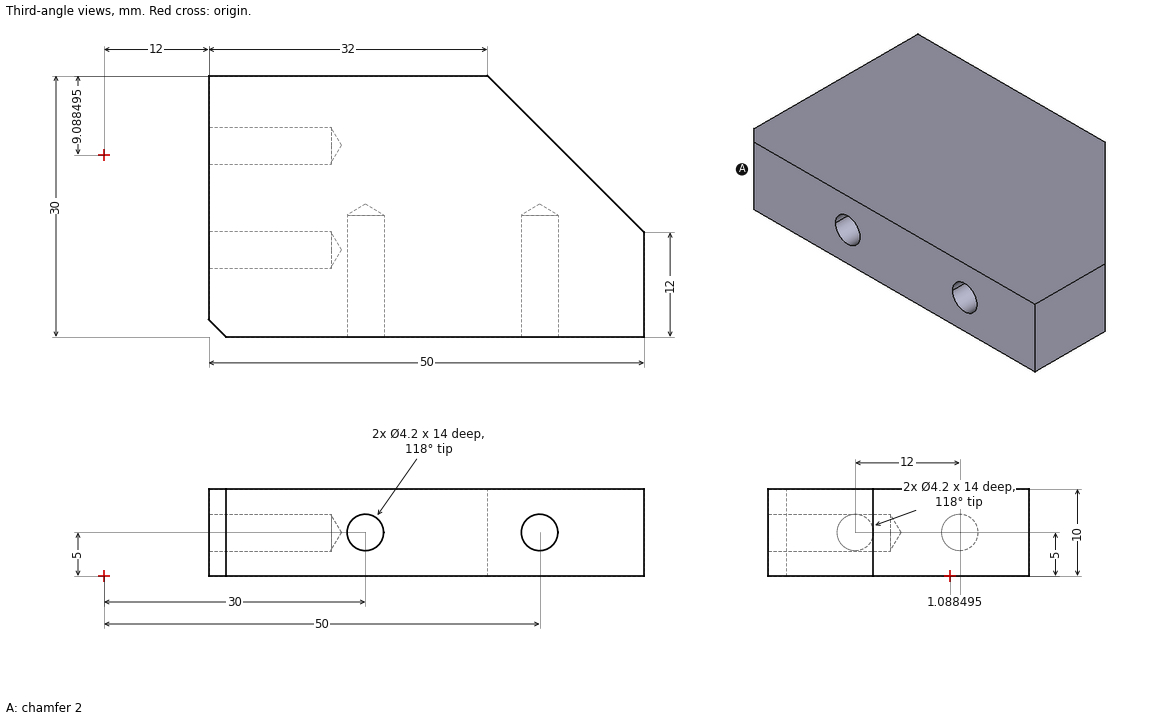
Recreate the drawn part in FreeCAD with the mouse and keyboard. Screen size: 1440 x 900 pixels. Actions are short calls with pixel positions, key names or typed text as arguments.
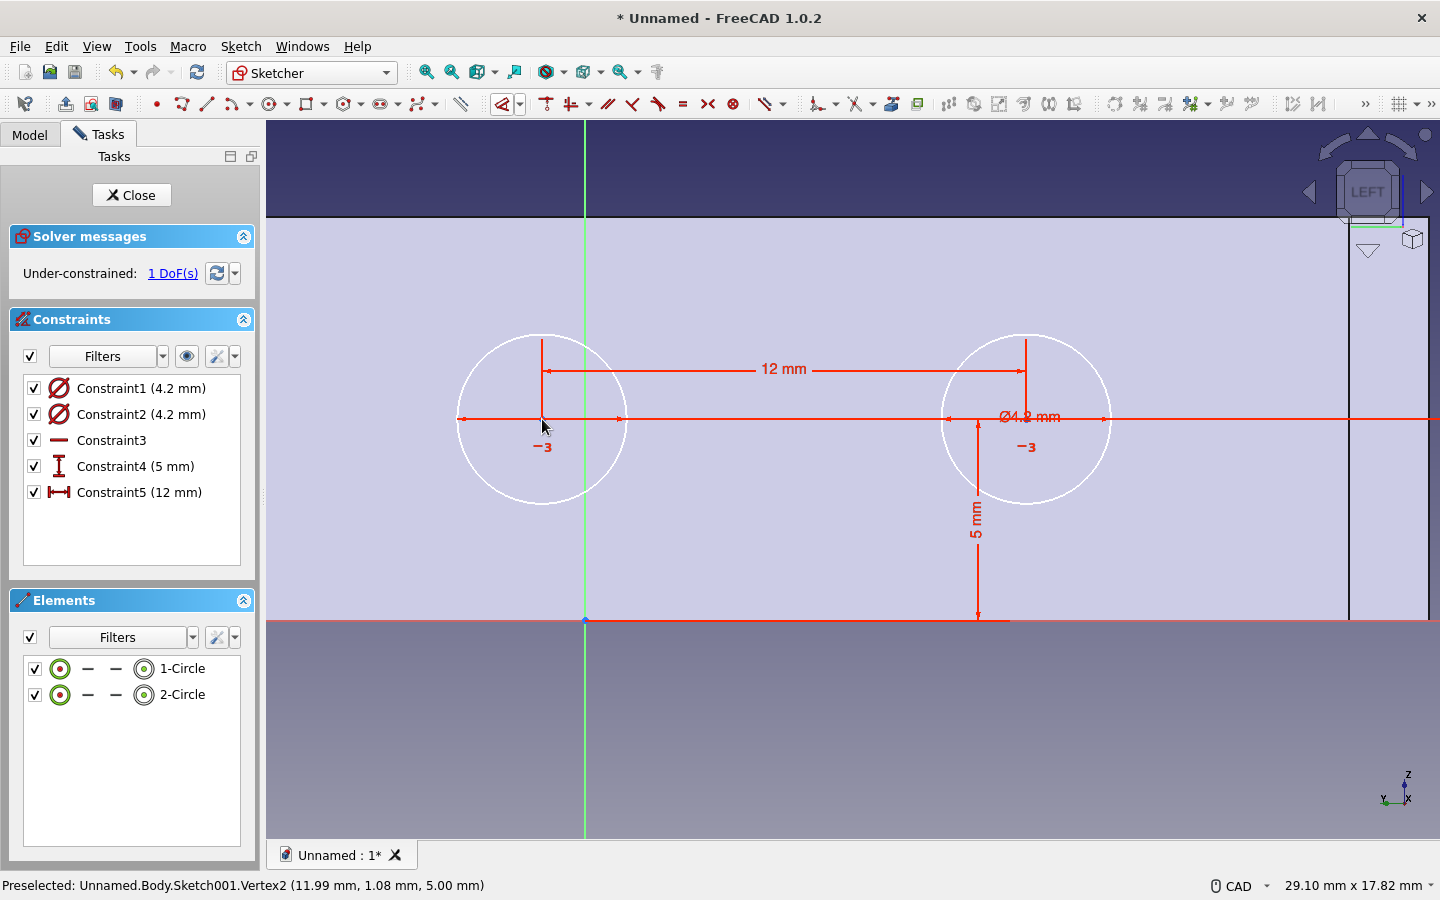
click(542, 419)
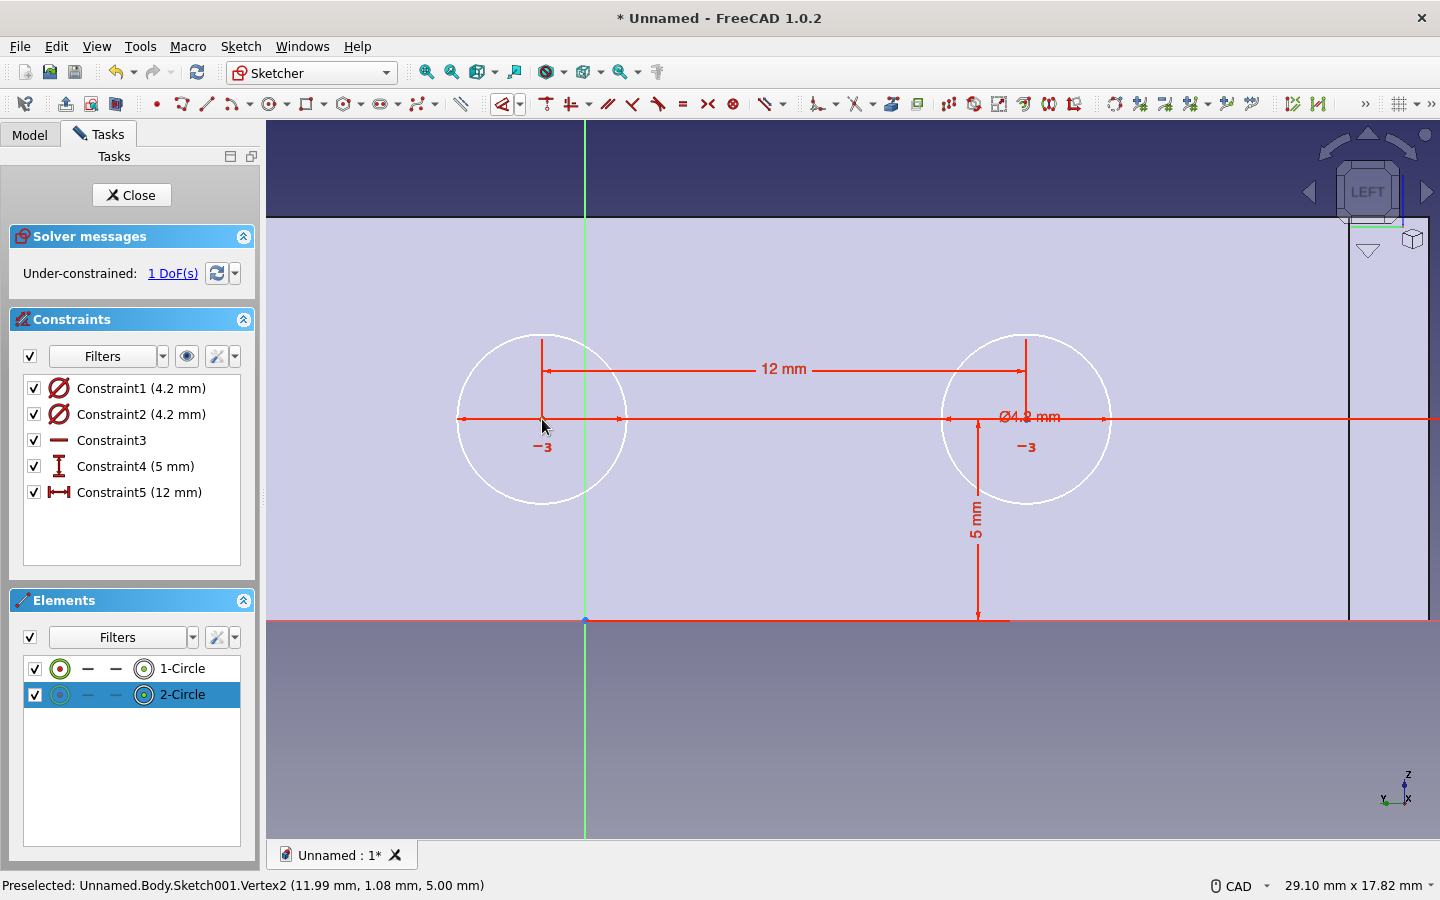
click(520, 104)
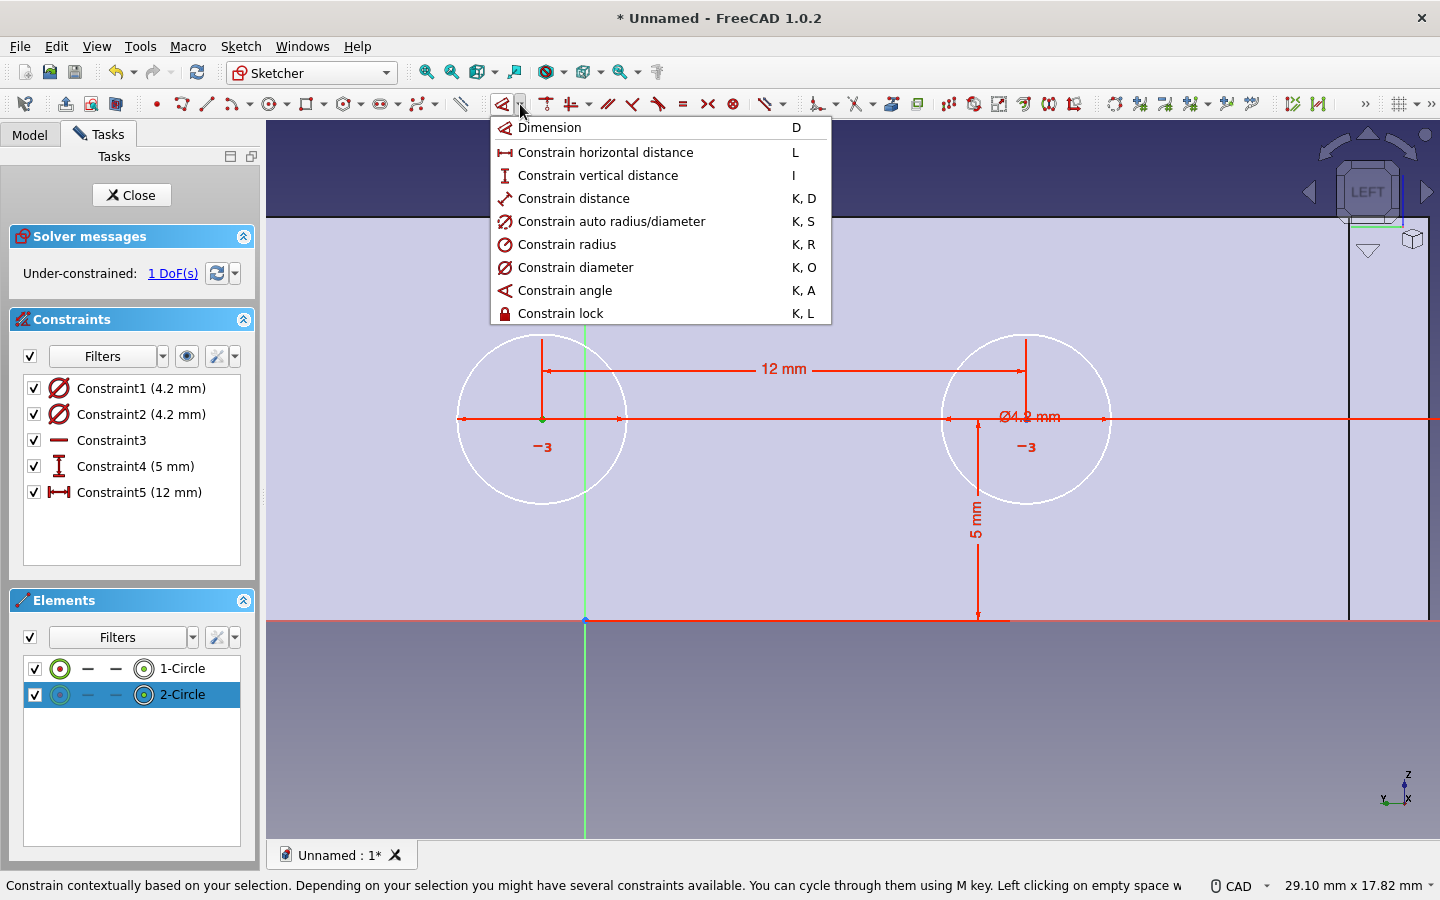
click(661, 152)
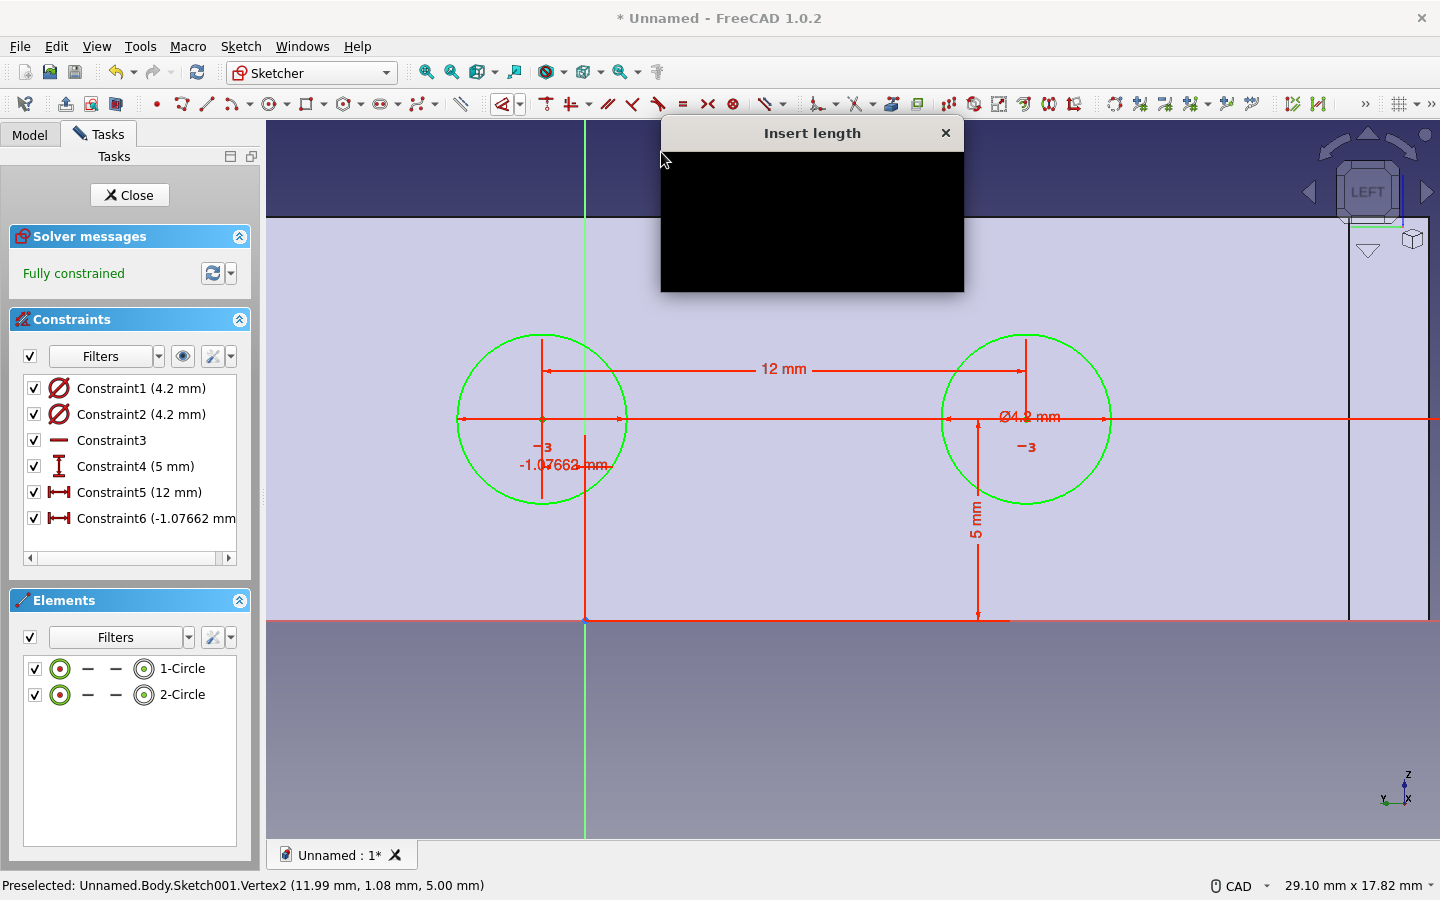
text(-1.088495)
key(Return)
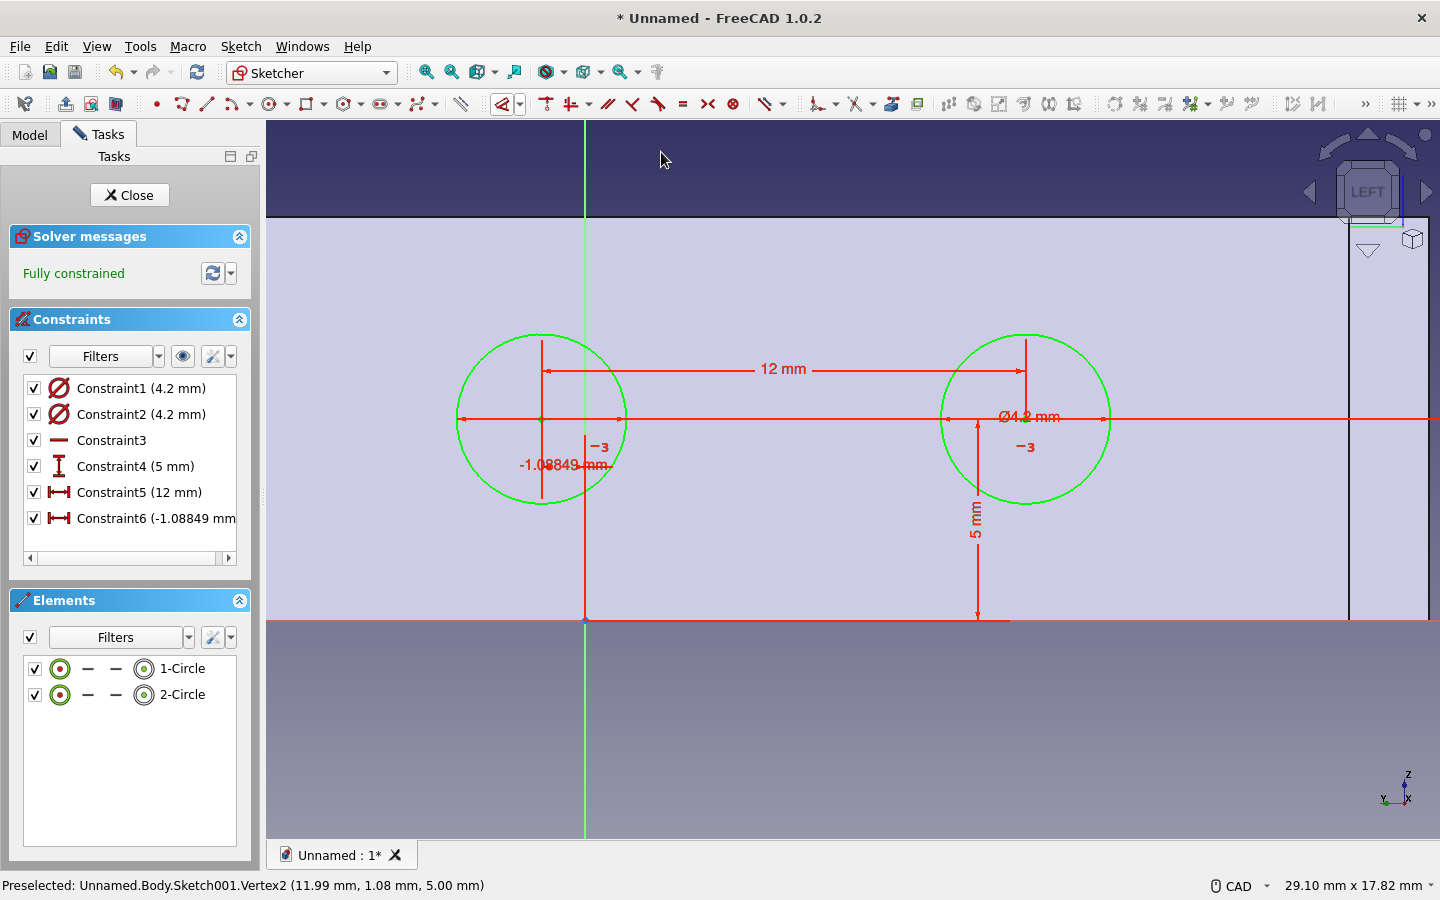
click(130, 195)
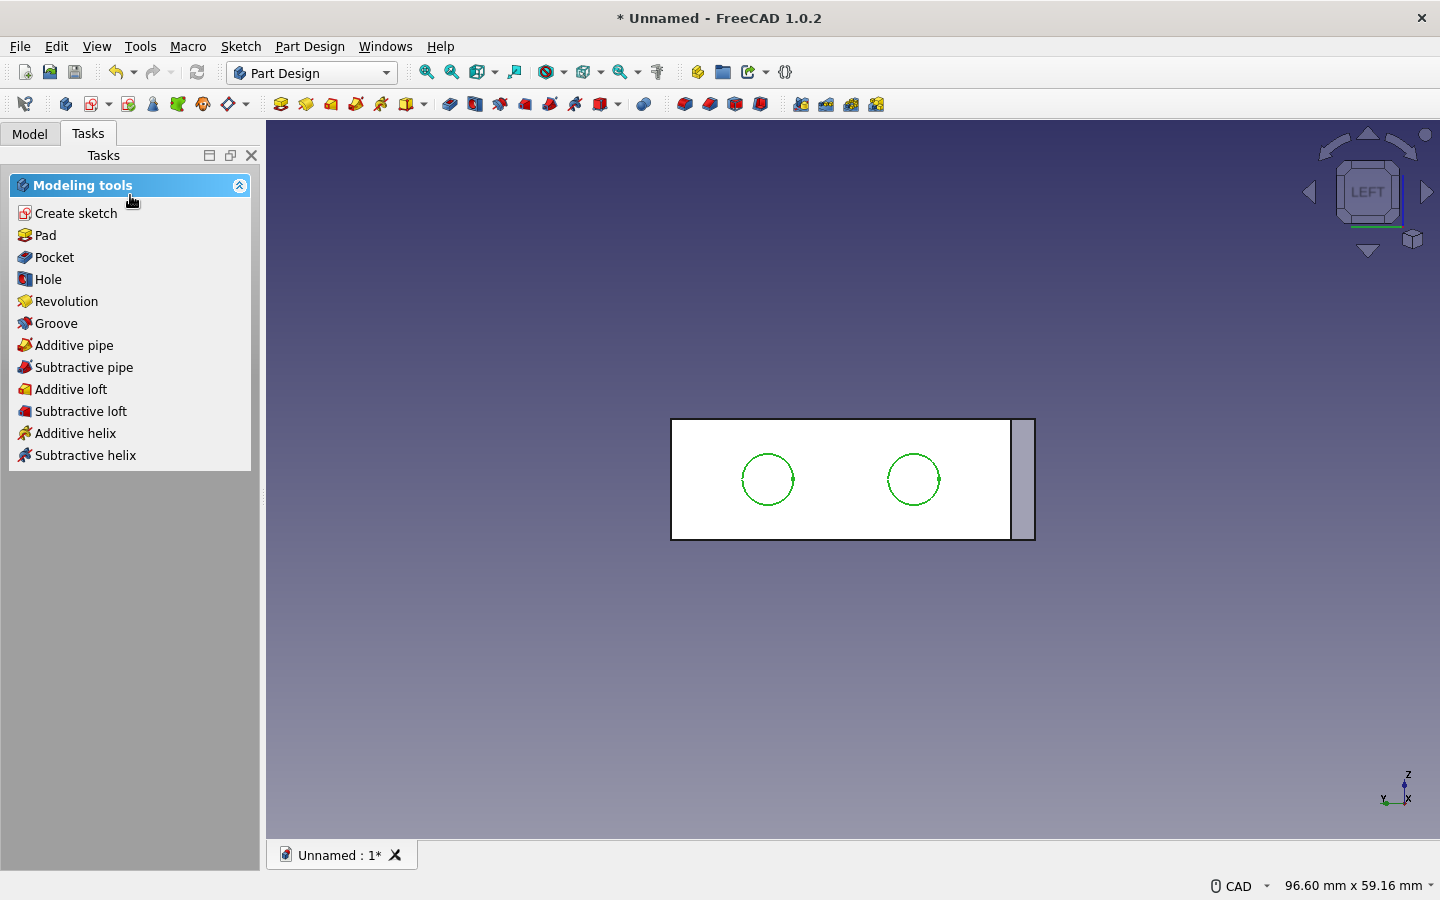
click(475, 104)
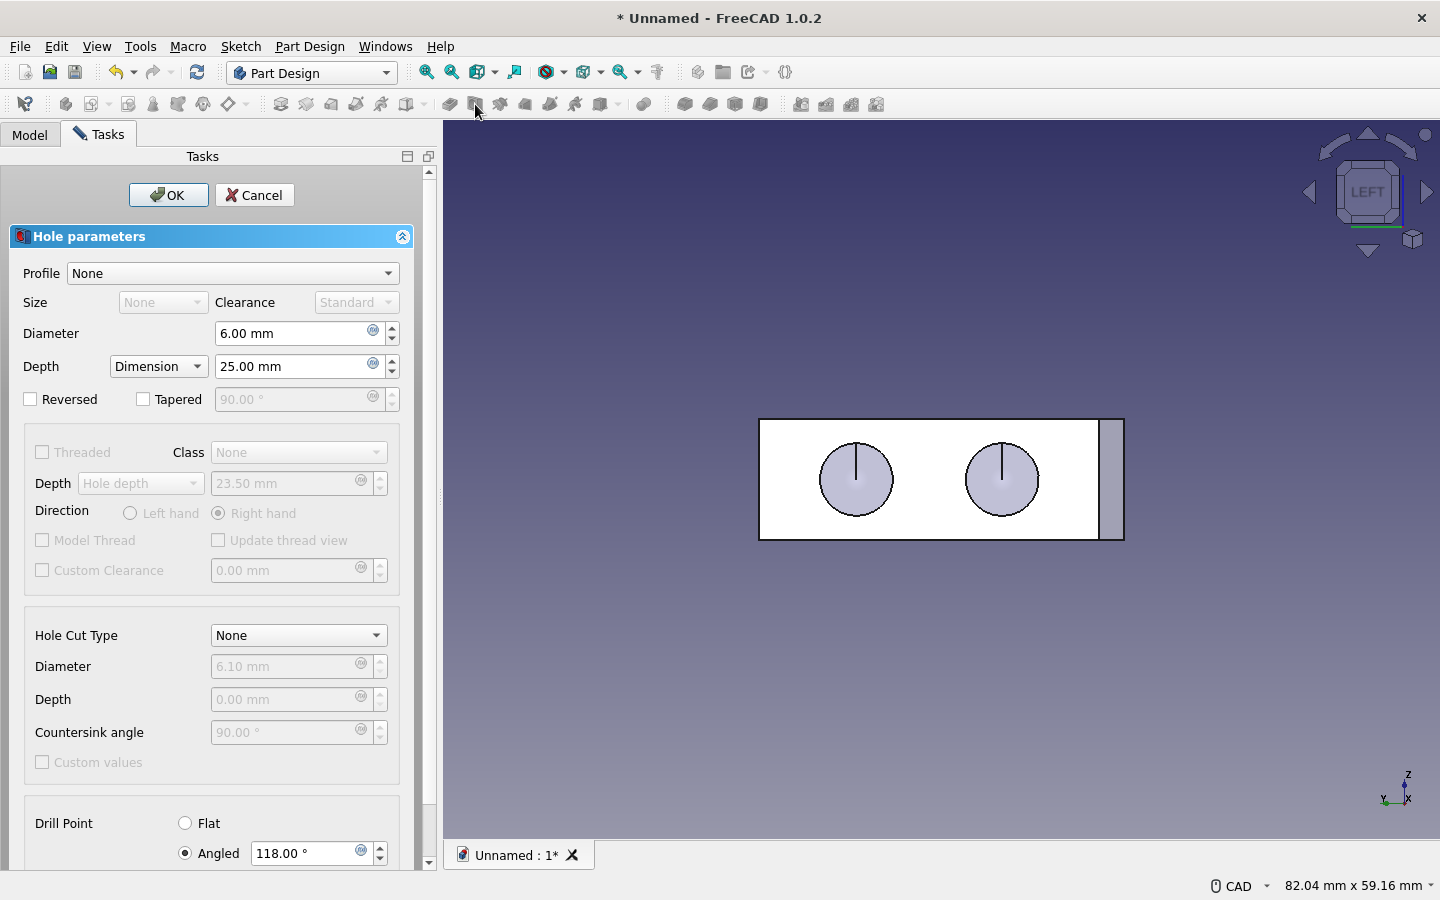
triple_click(300, 334)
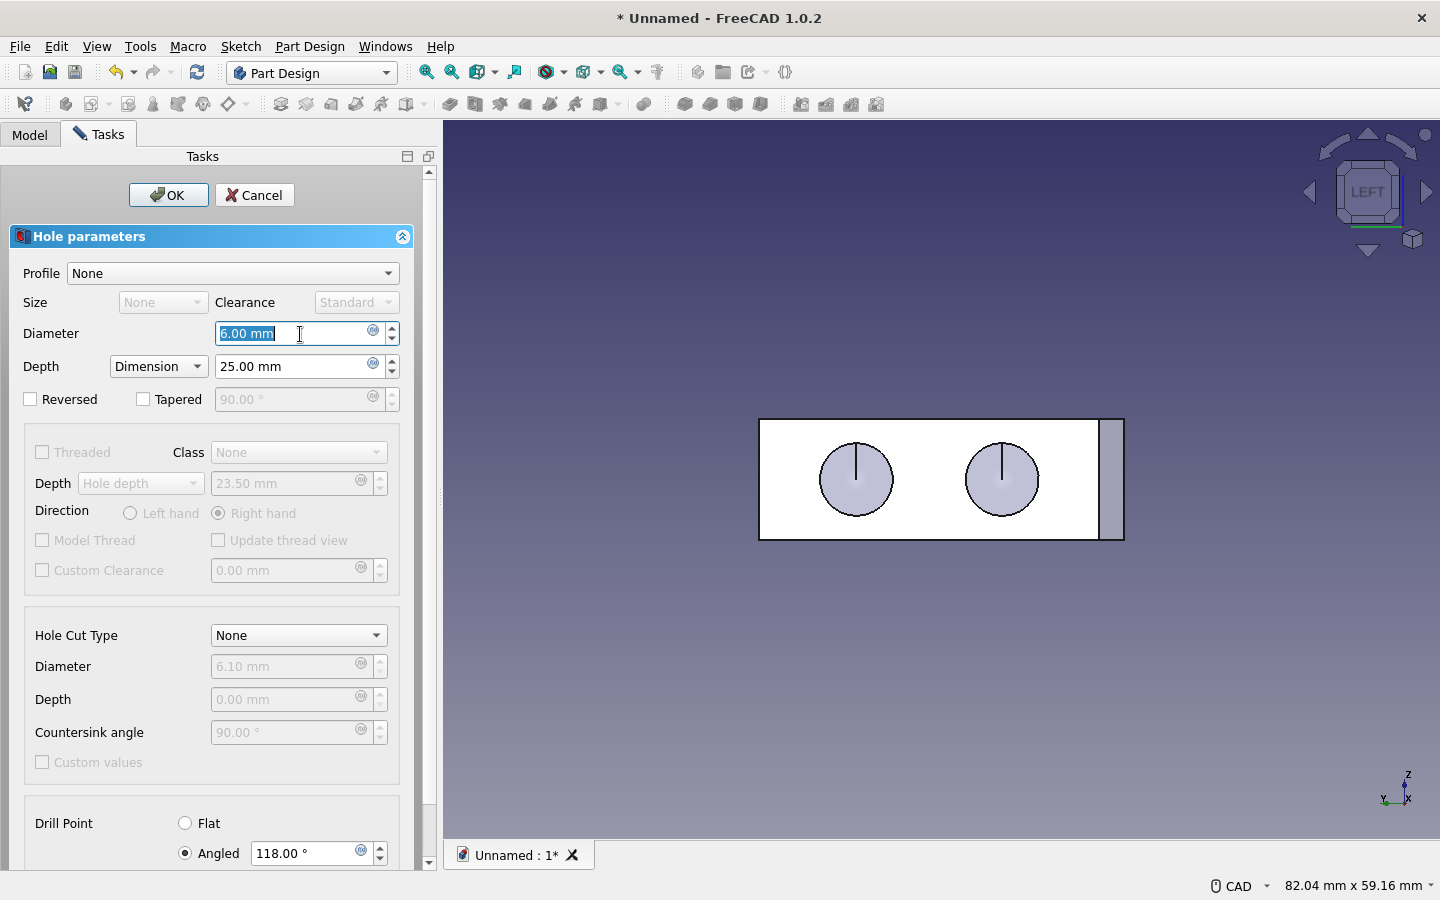
text(4.2)
key(Tab)